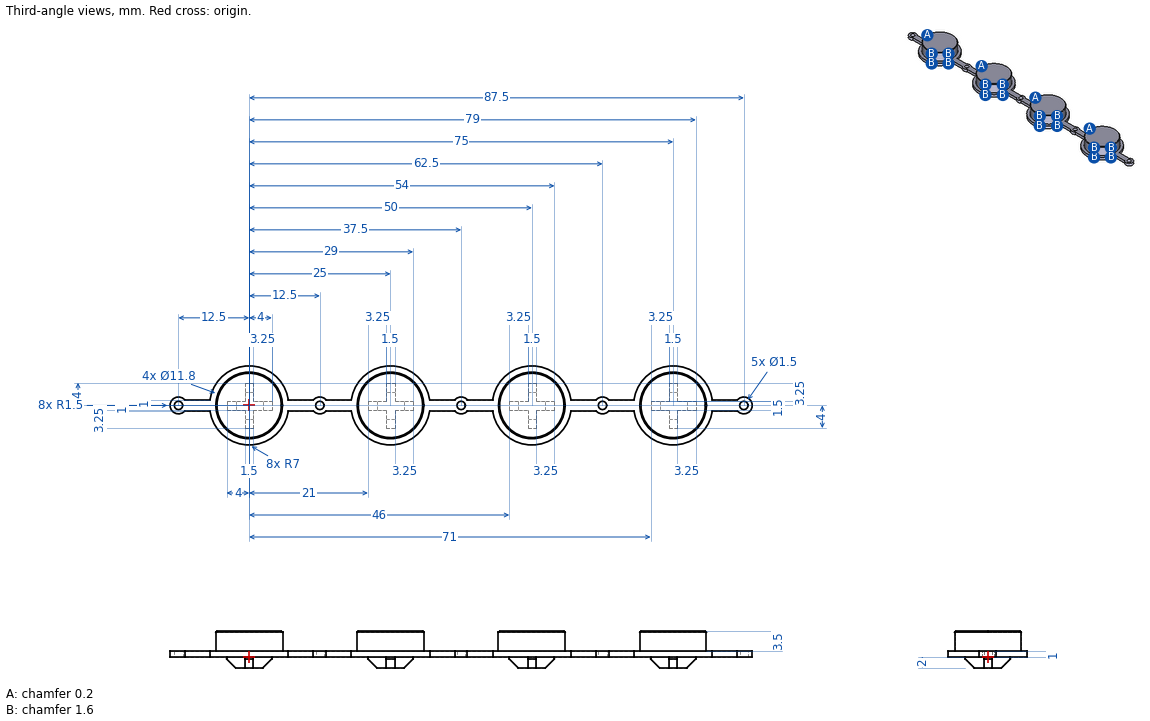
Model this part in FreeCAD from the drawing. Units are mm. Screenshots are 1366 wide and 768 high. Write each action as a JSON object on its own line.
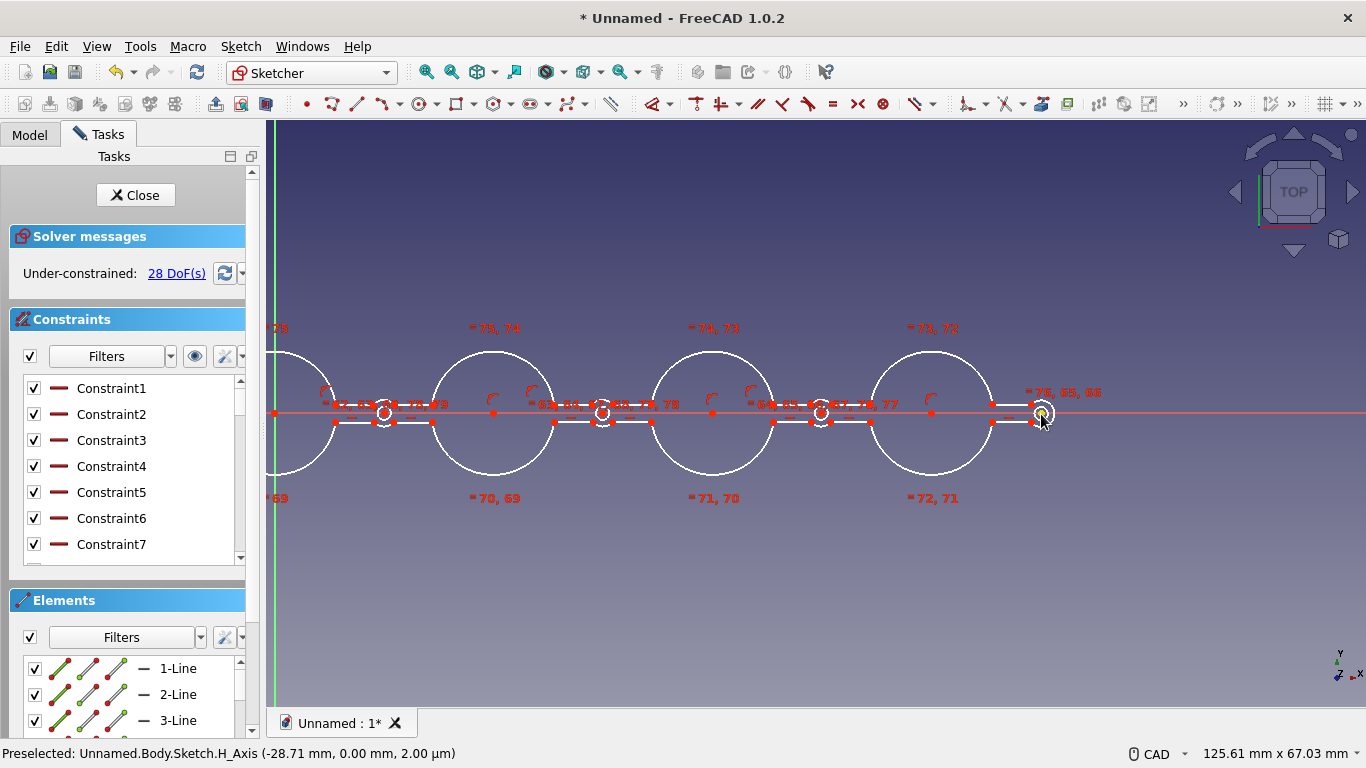
{"action": "left_click", "coordinate": [1041, 414]}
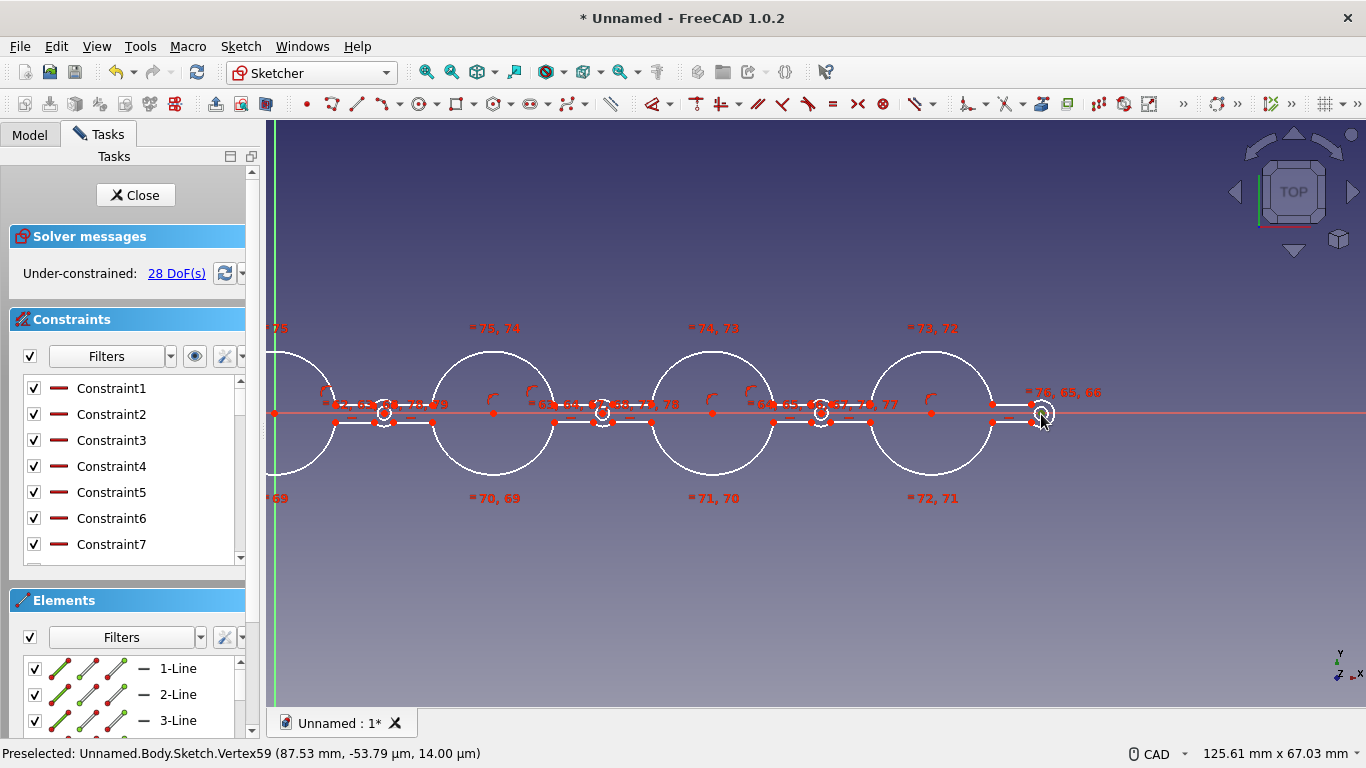
{"action": "left_click", "coordinate": [488, 413]}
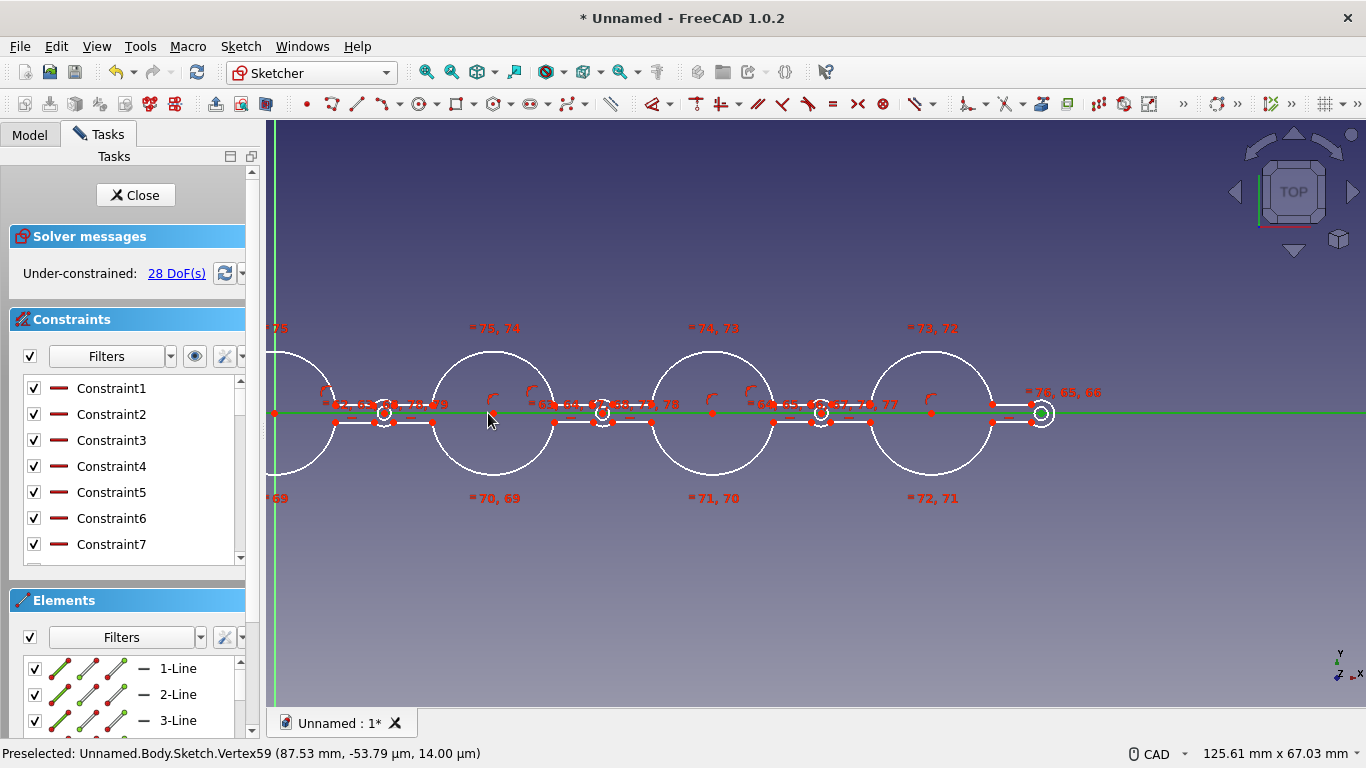
{"action": "key", "text": "c"}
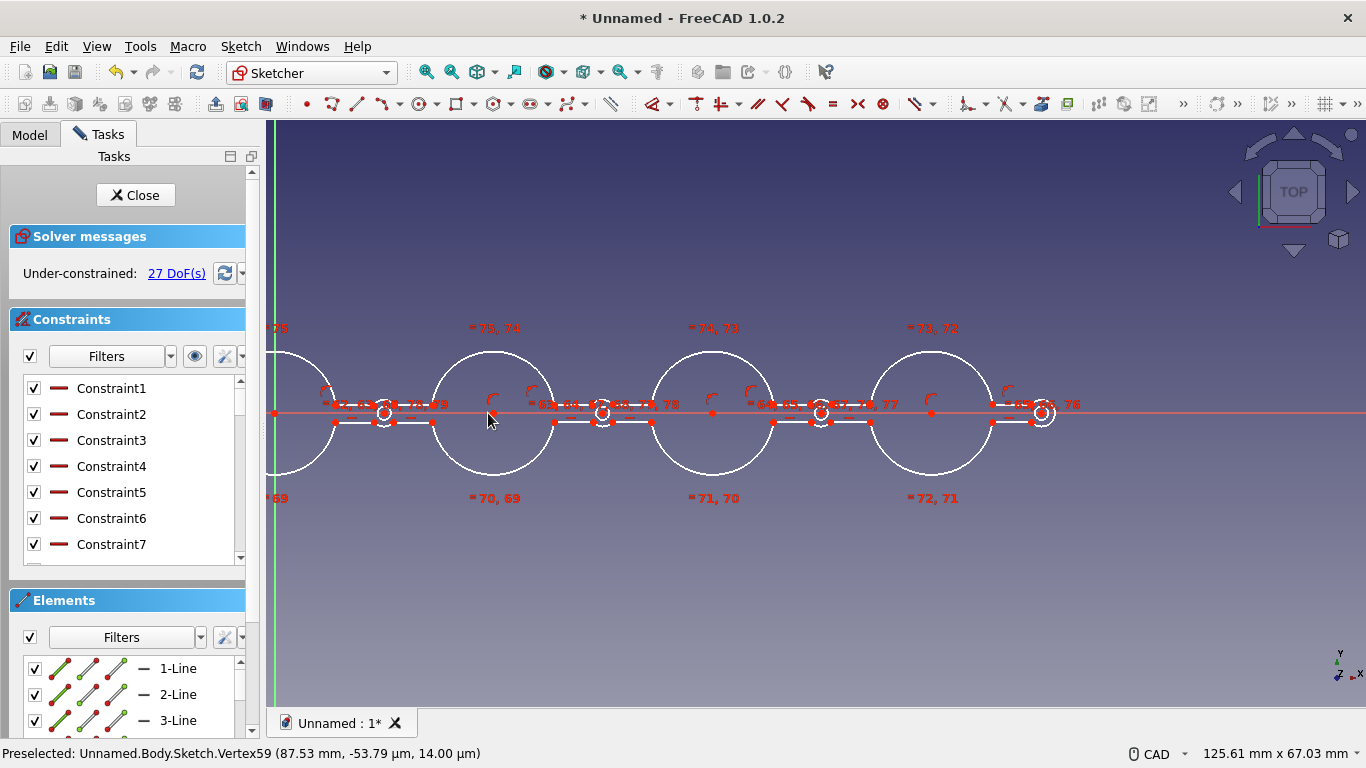
{"action": "key", "text": "d"}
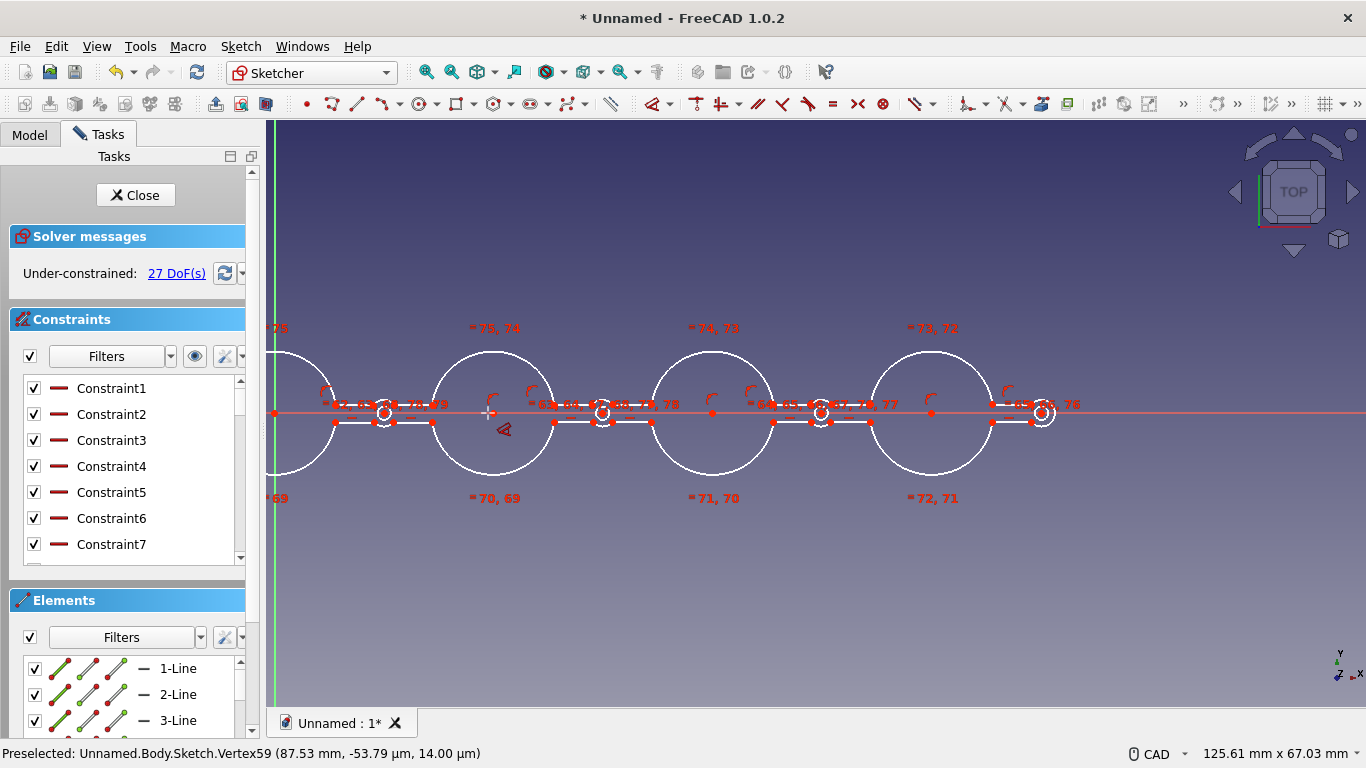
{"action": "scroll", "coordinate": [1041, 414], "scroll_direction": "down", "scroll_amount": 2}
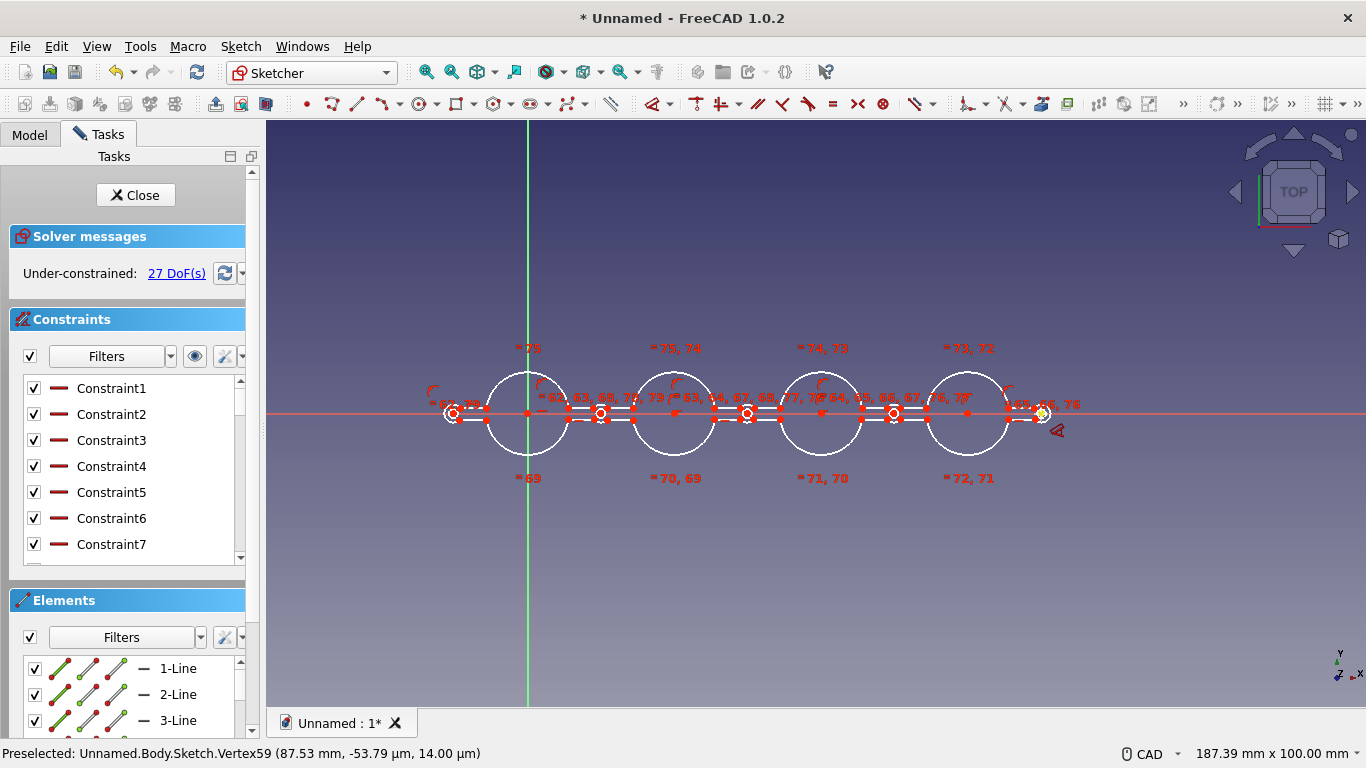
{"action": "scroll", "coordinate": [448, 421], "scroll_direction": "up", "scroll_amount": 8}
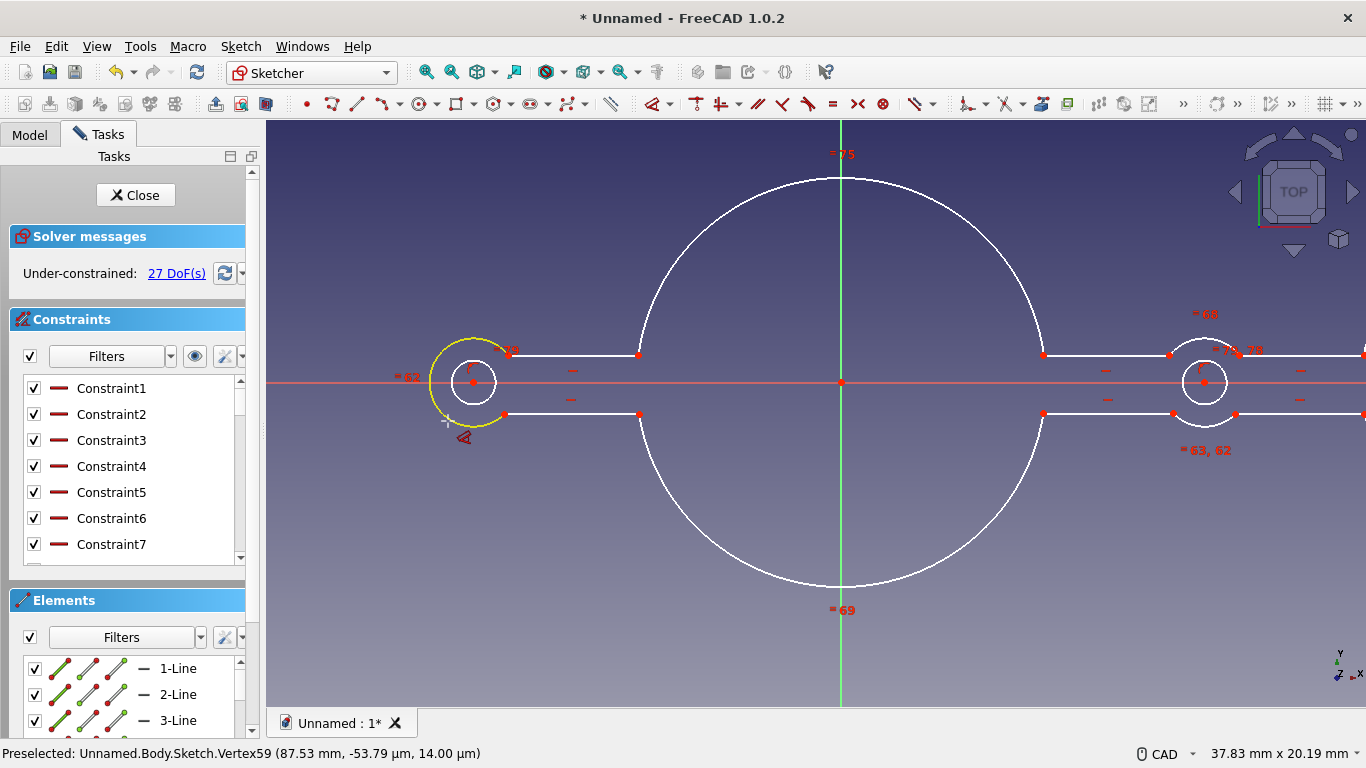
{"action": "left_click", "coordinate": [446, 417]}
{"action": "left_click", "coordinate": [426, 442]}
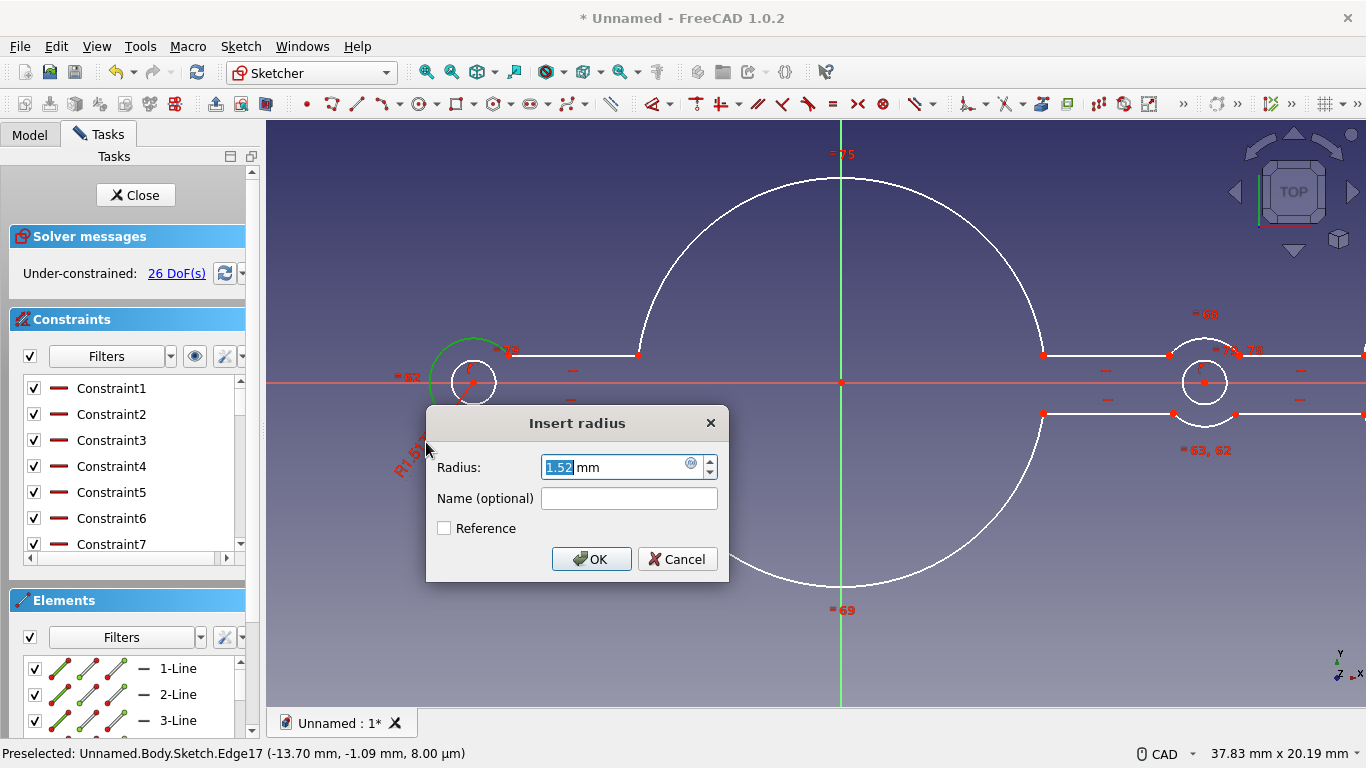
{"action": "type", "text": "1.5"}
{"action": "key", "text": "Return"}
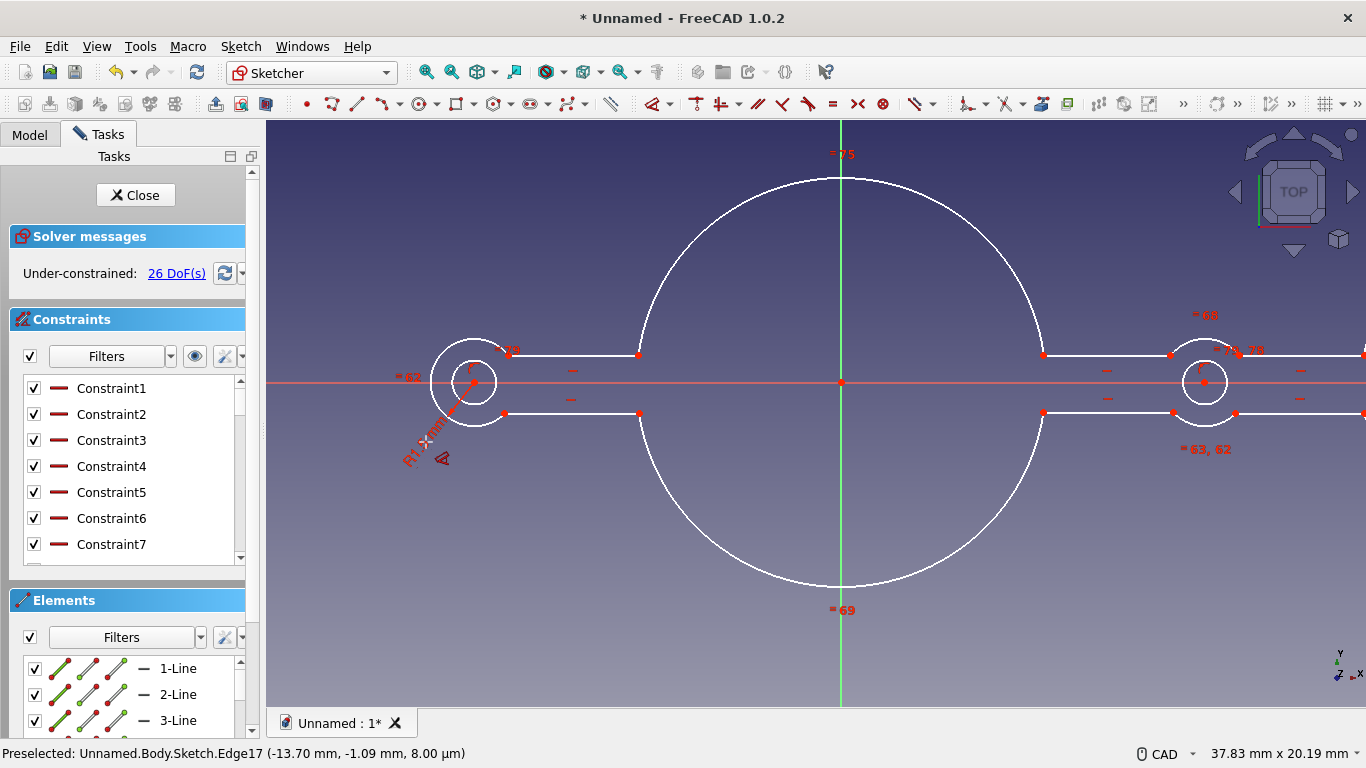
{"action": "scroll", "coordinate": [448, 421], "scroll_direction": "down", "scroll_amount": 8}